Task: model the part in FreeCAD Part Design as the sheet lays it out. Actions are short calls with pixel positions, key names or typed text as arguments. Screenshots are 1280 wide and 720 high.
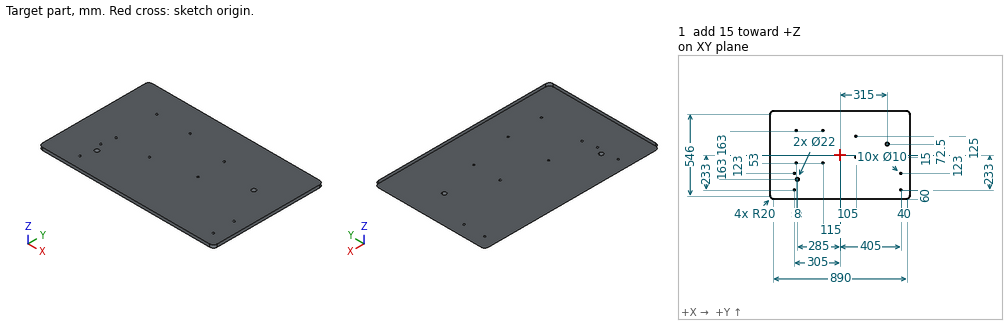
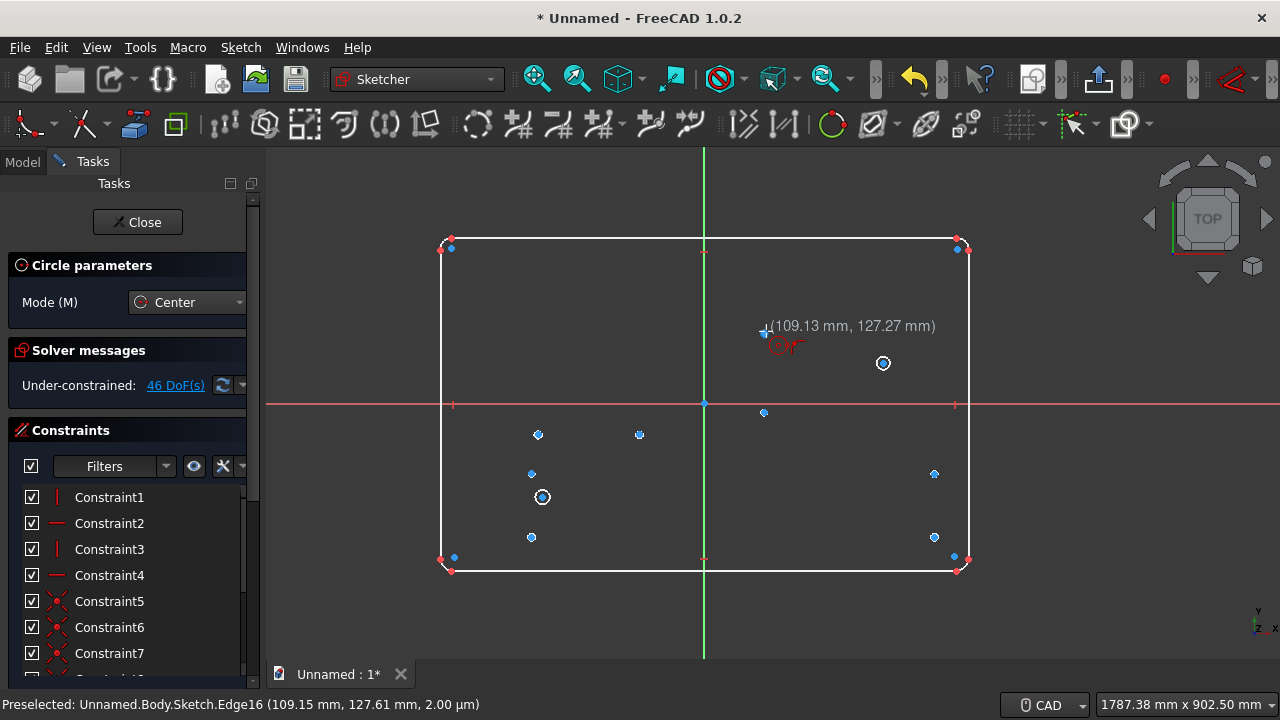
scroll(639, 311, up, 11)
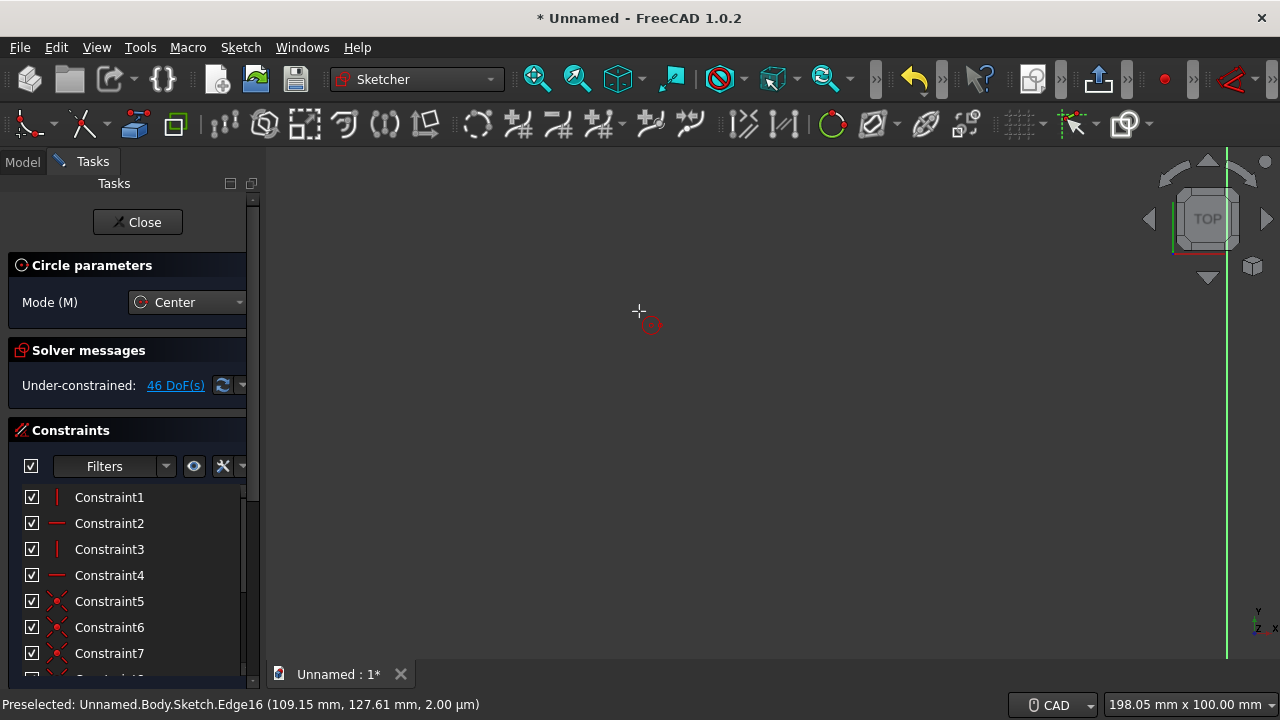
scroll(639, 311, down, 11)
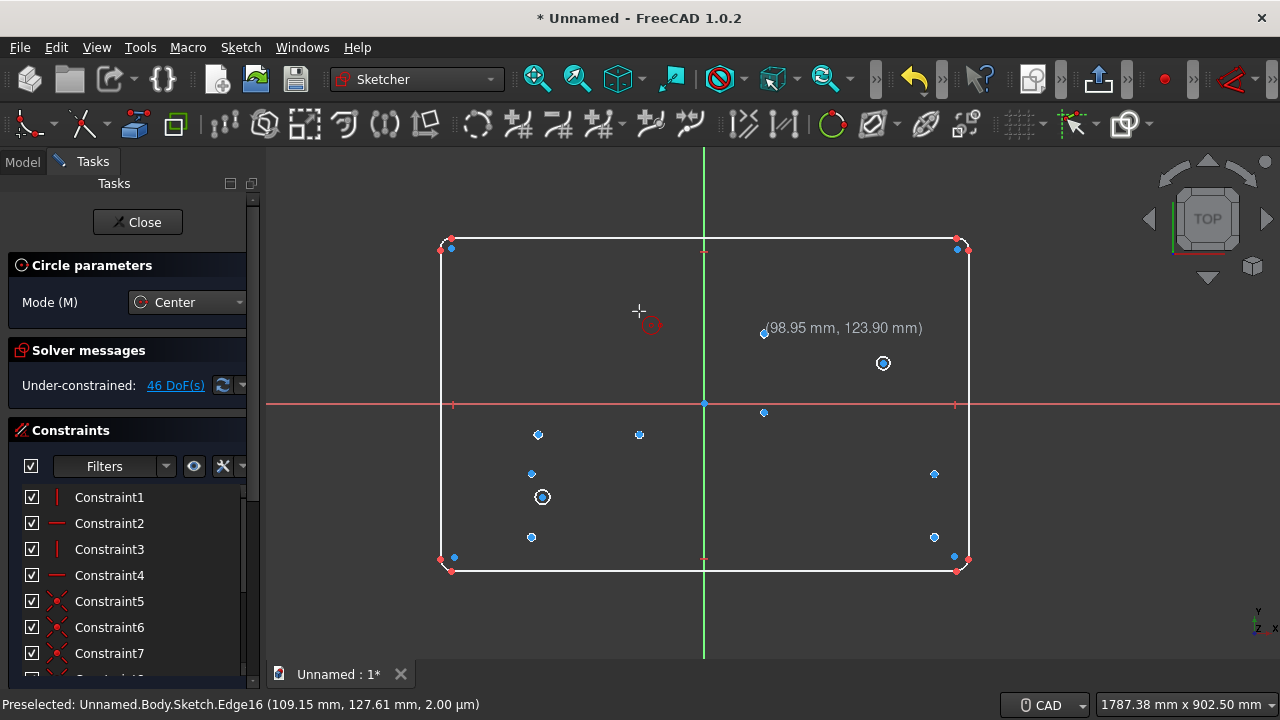
click(639, 311)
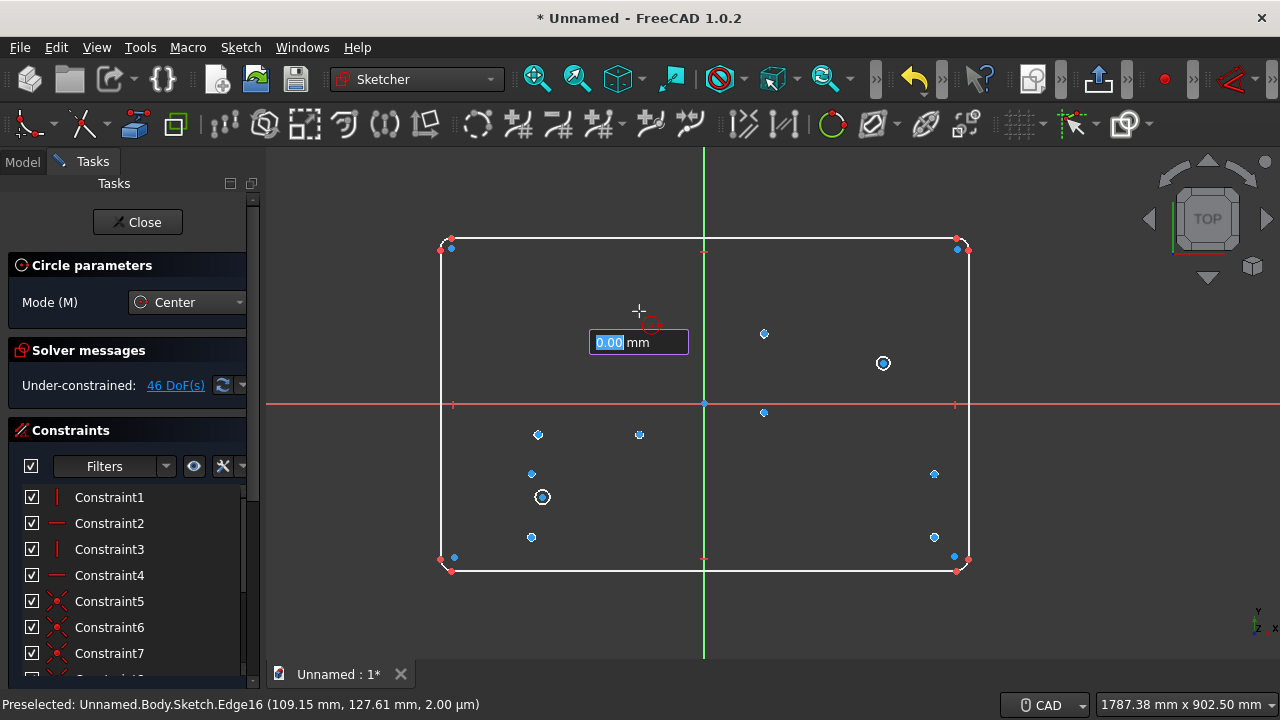
scroll(641, 309, up, 9)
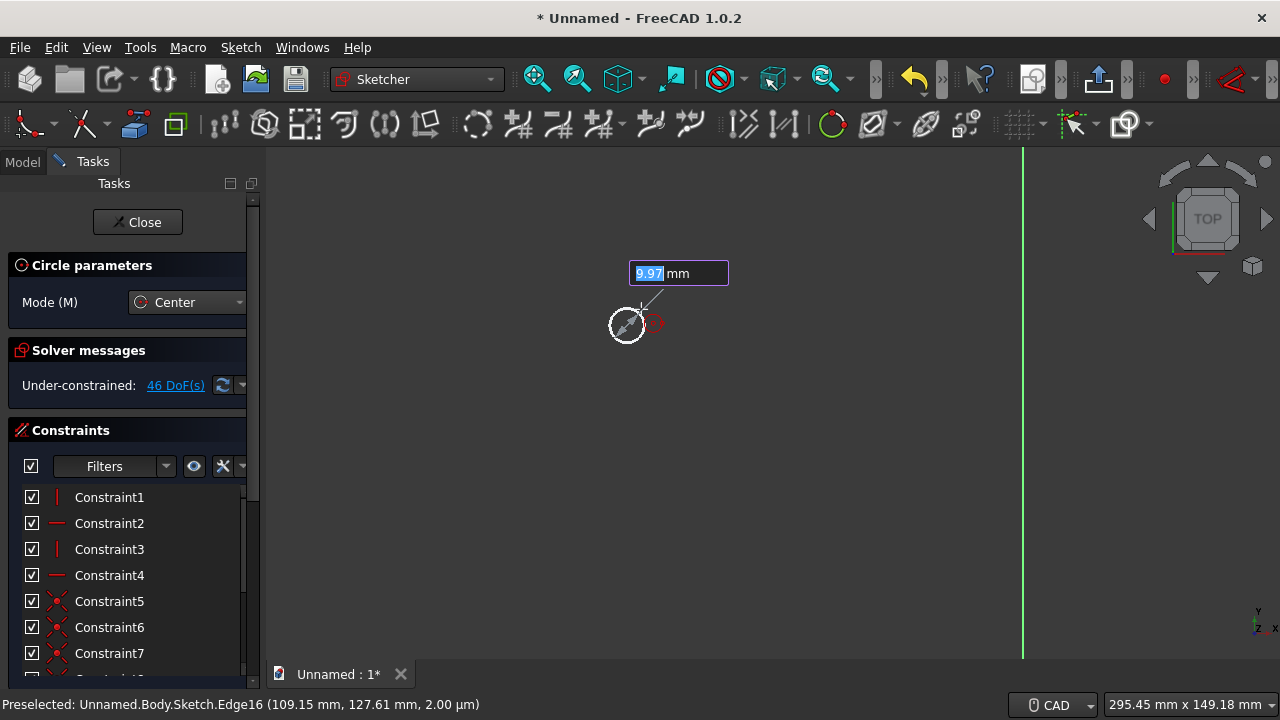
click(641, 309)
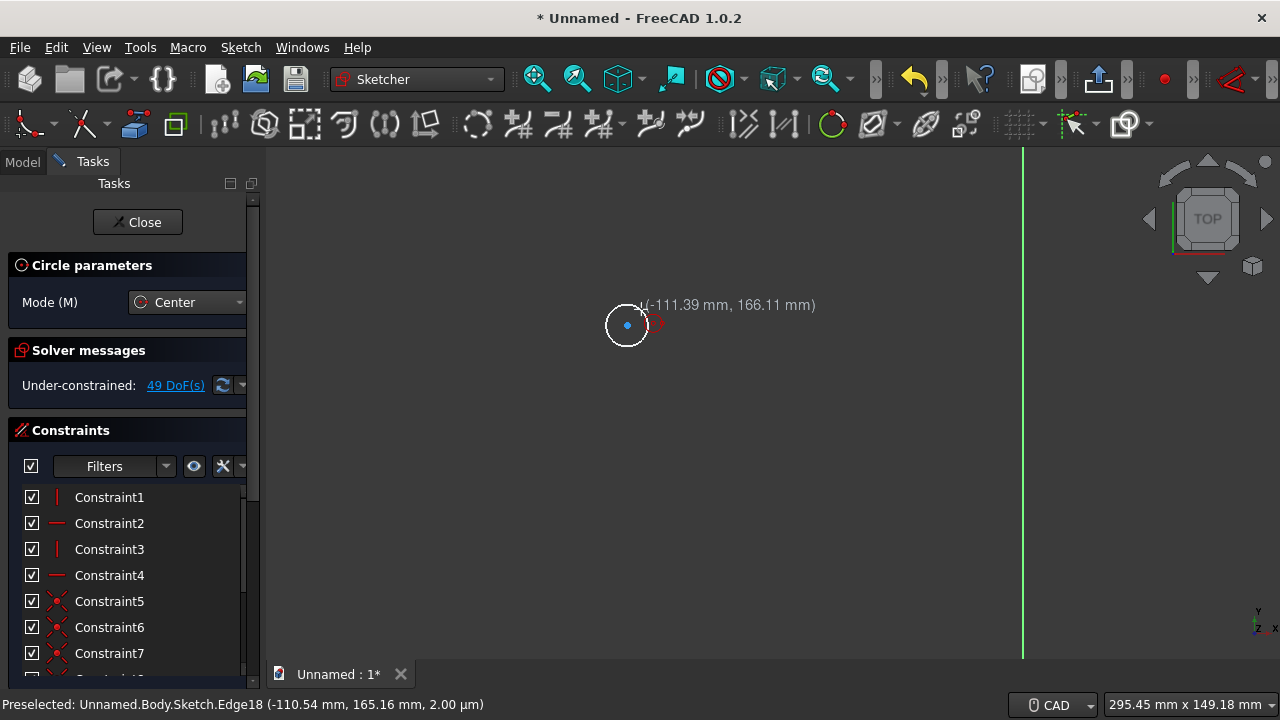
scroll(641, 309, down, 9)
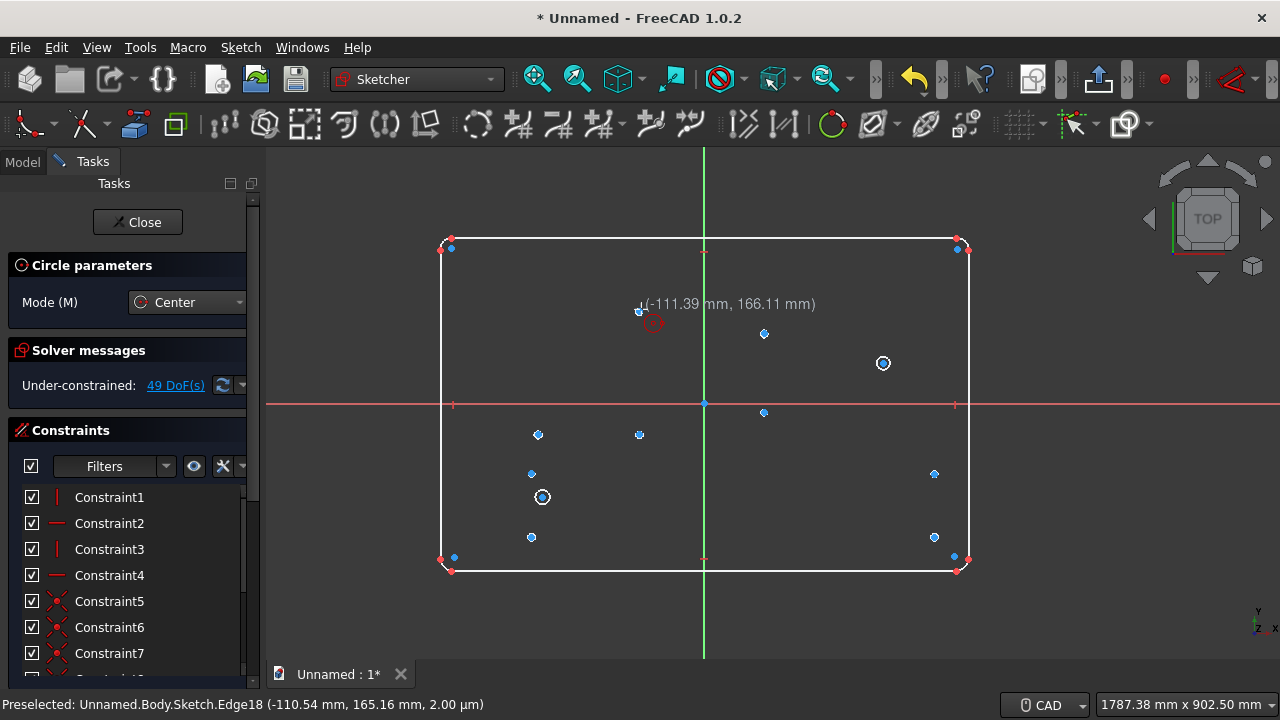
scroll(538, 311, up, 11)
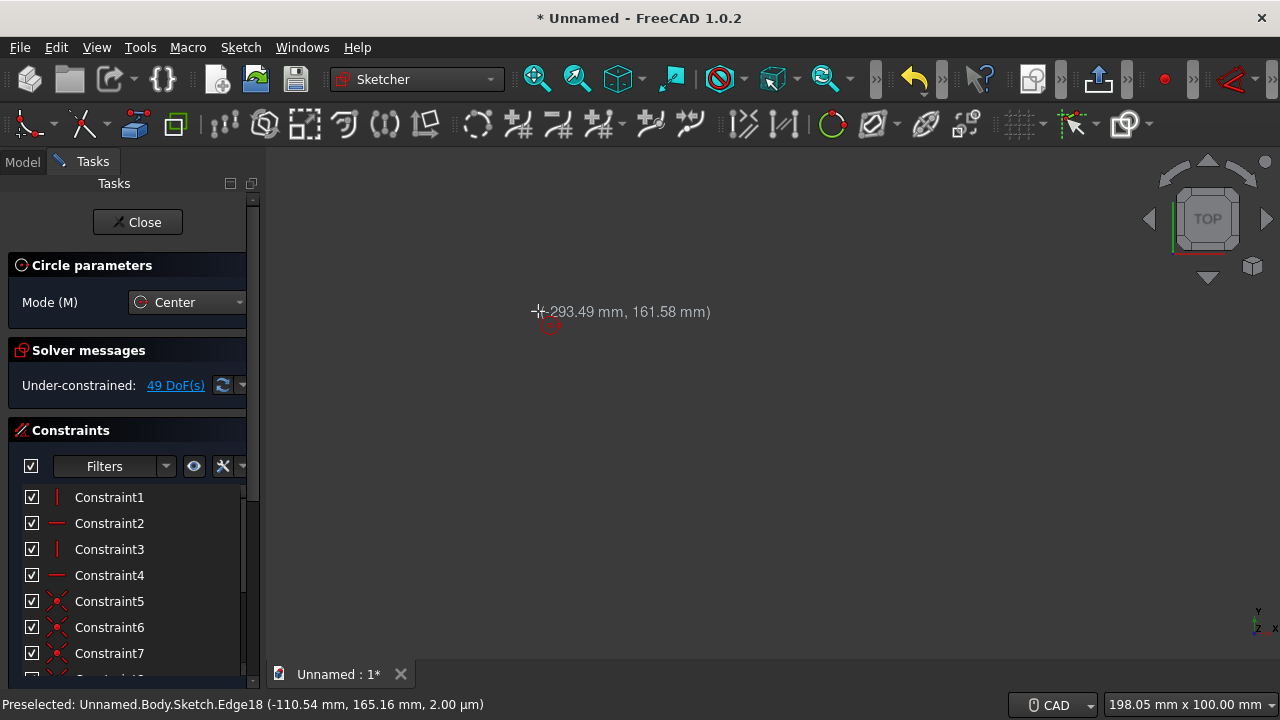
scroll(538, 311, down, 11)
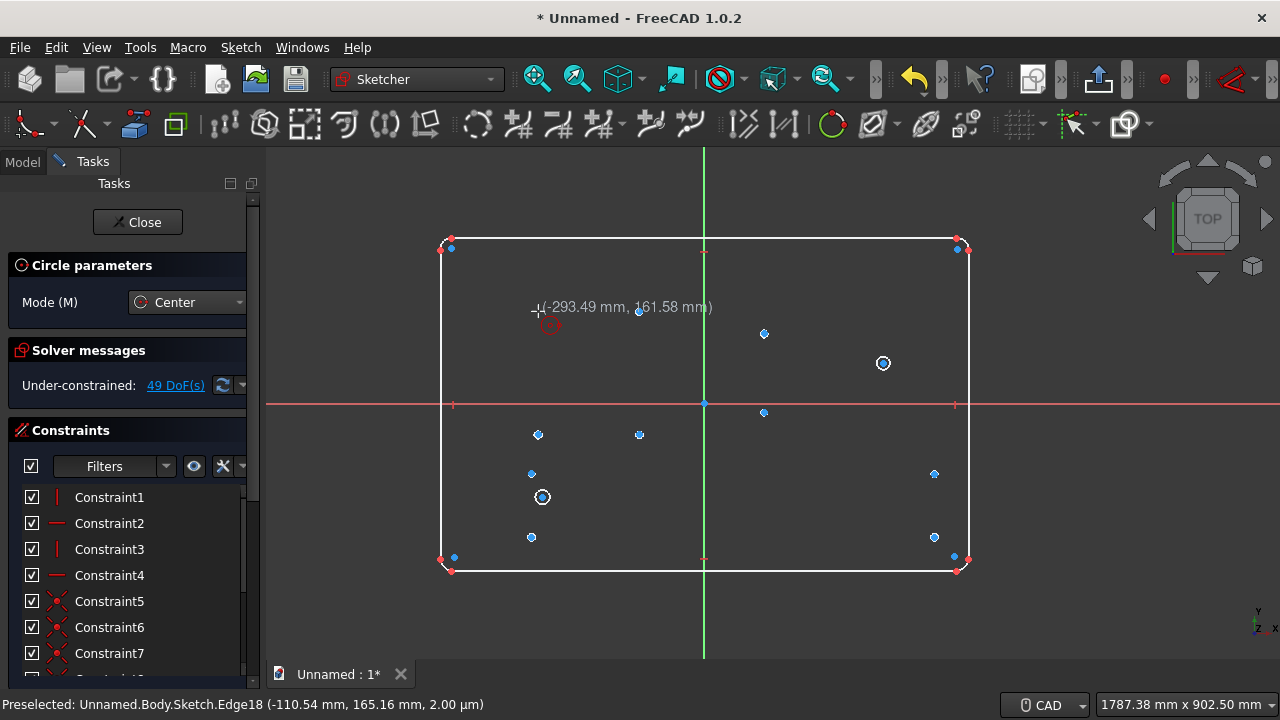
click(538, 311)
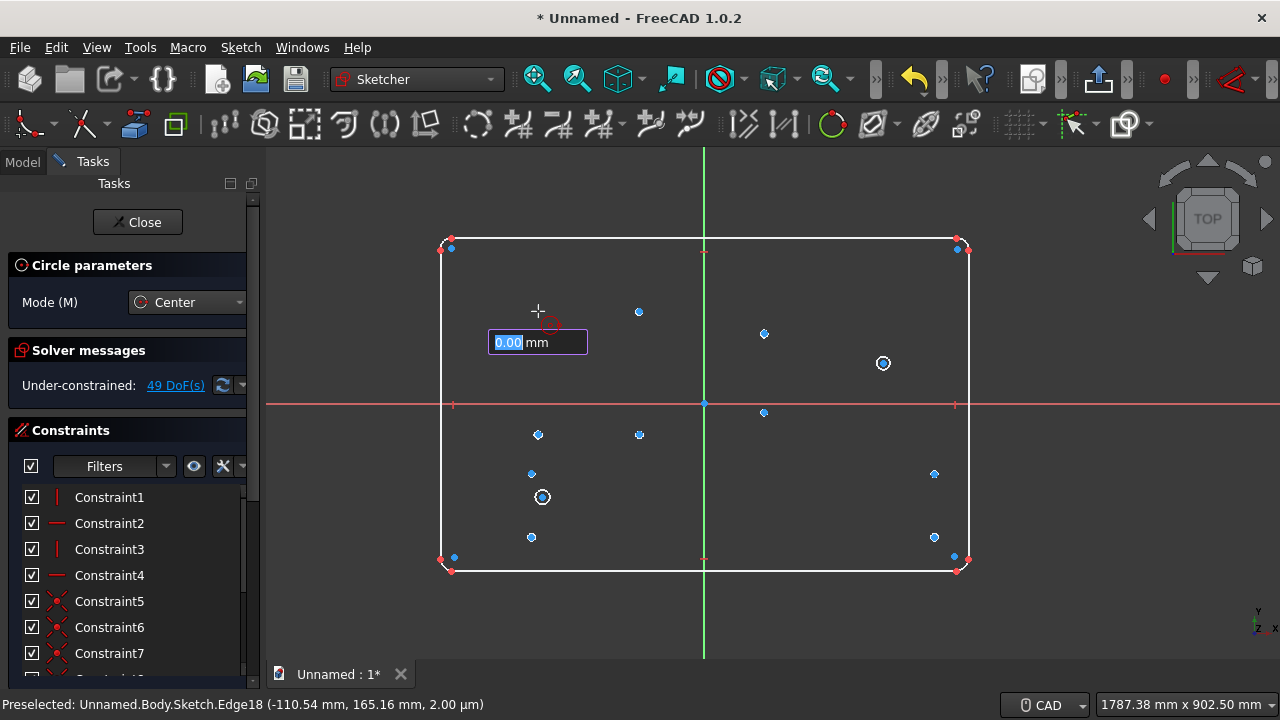
scroll(540, 309, up, 9)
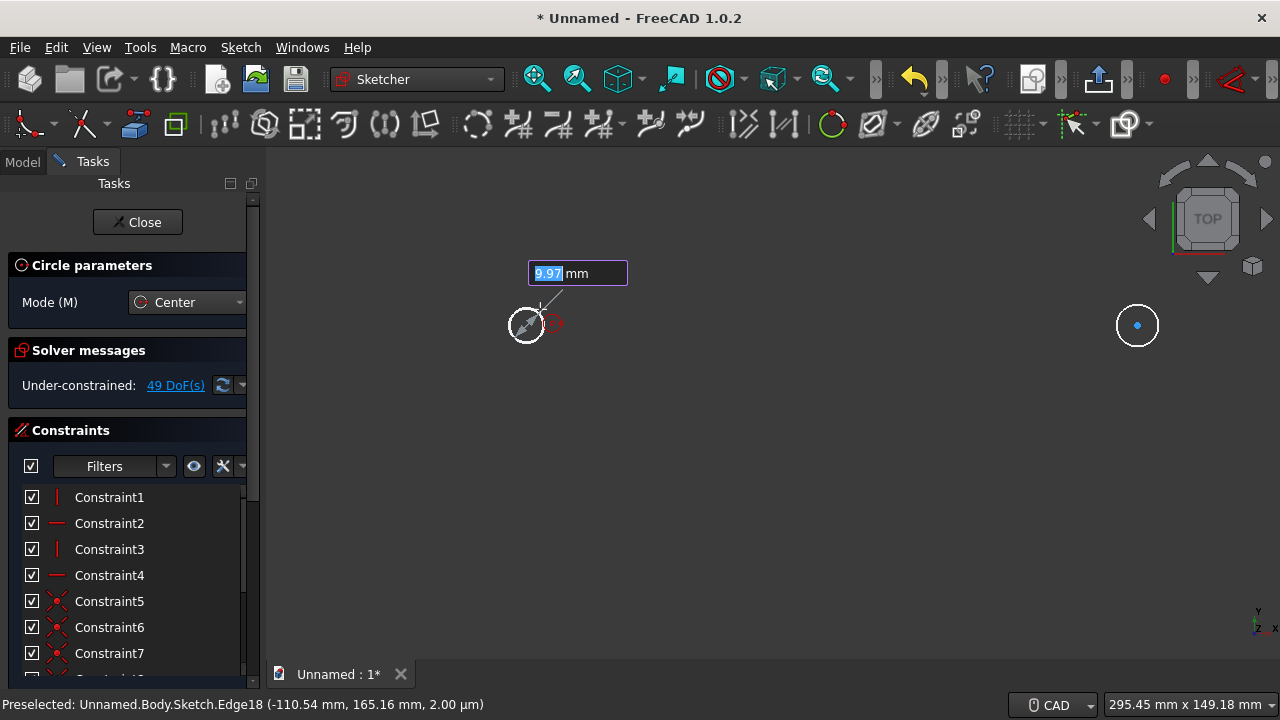
click(540, 309)
key(Escape)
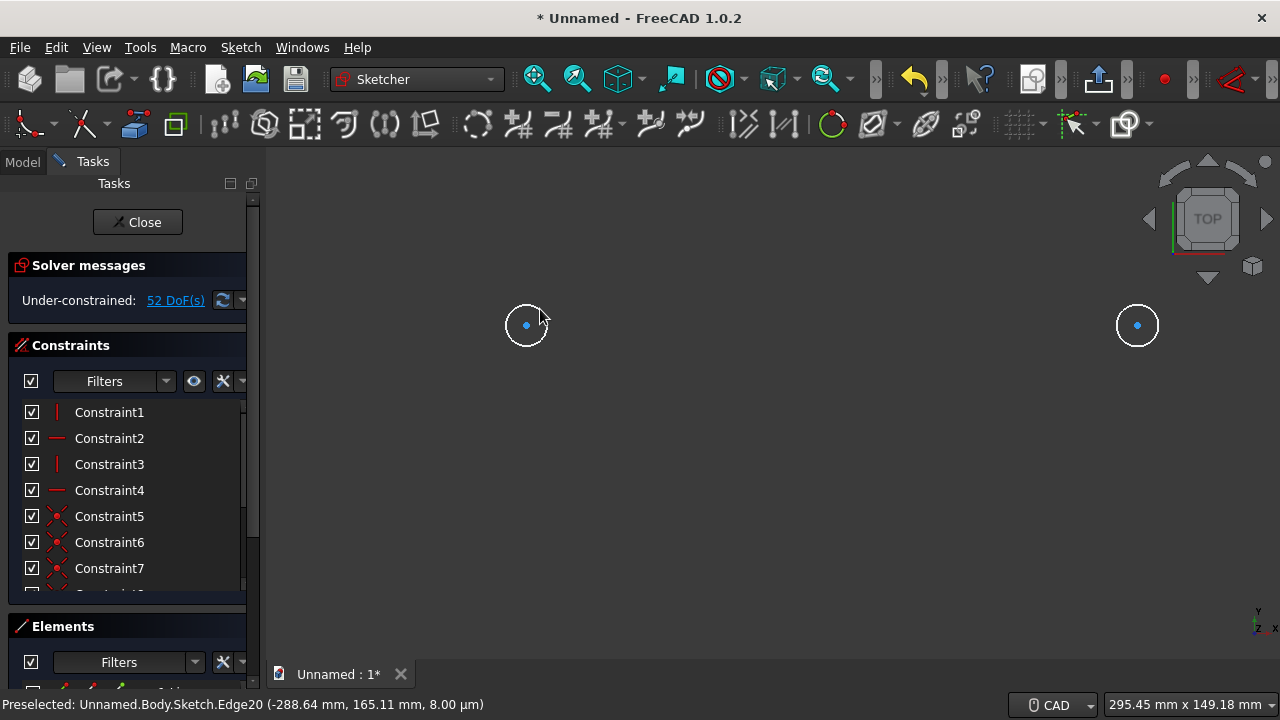
scroll(540, 309, down, 9)